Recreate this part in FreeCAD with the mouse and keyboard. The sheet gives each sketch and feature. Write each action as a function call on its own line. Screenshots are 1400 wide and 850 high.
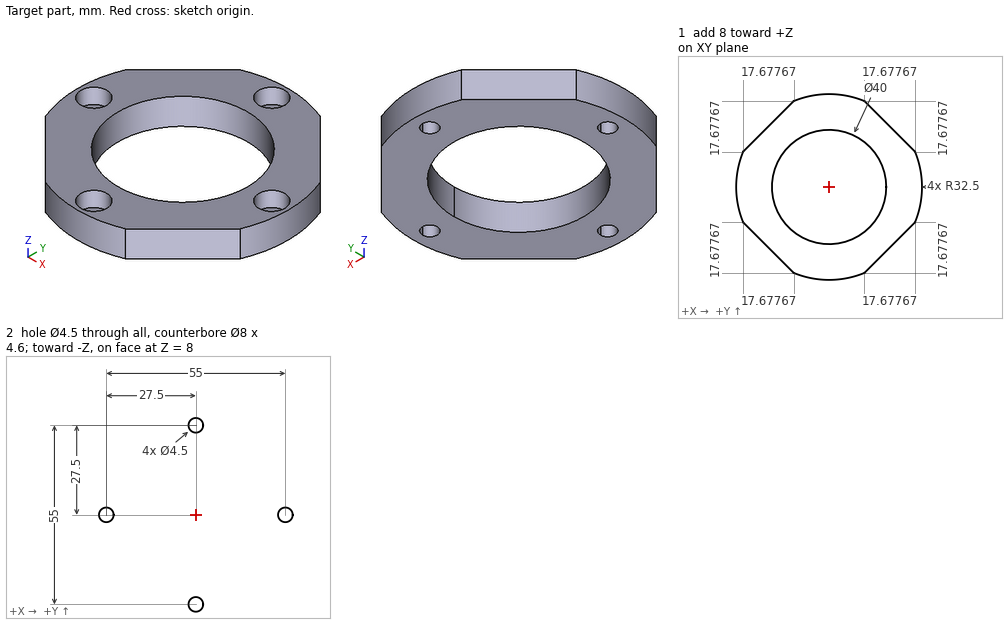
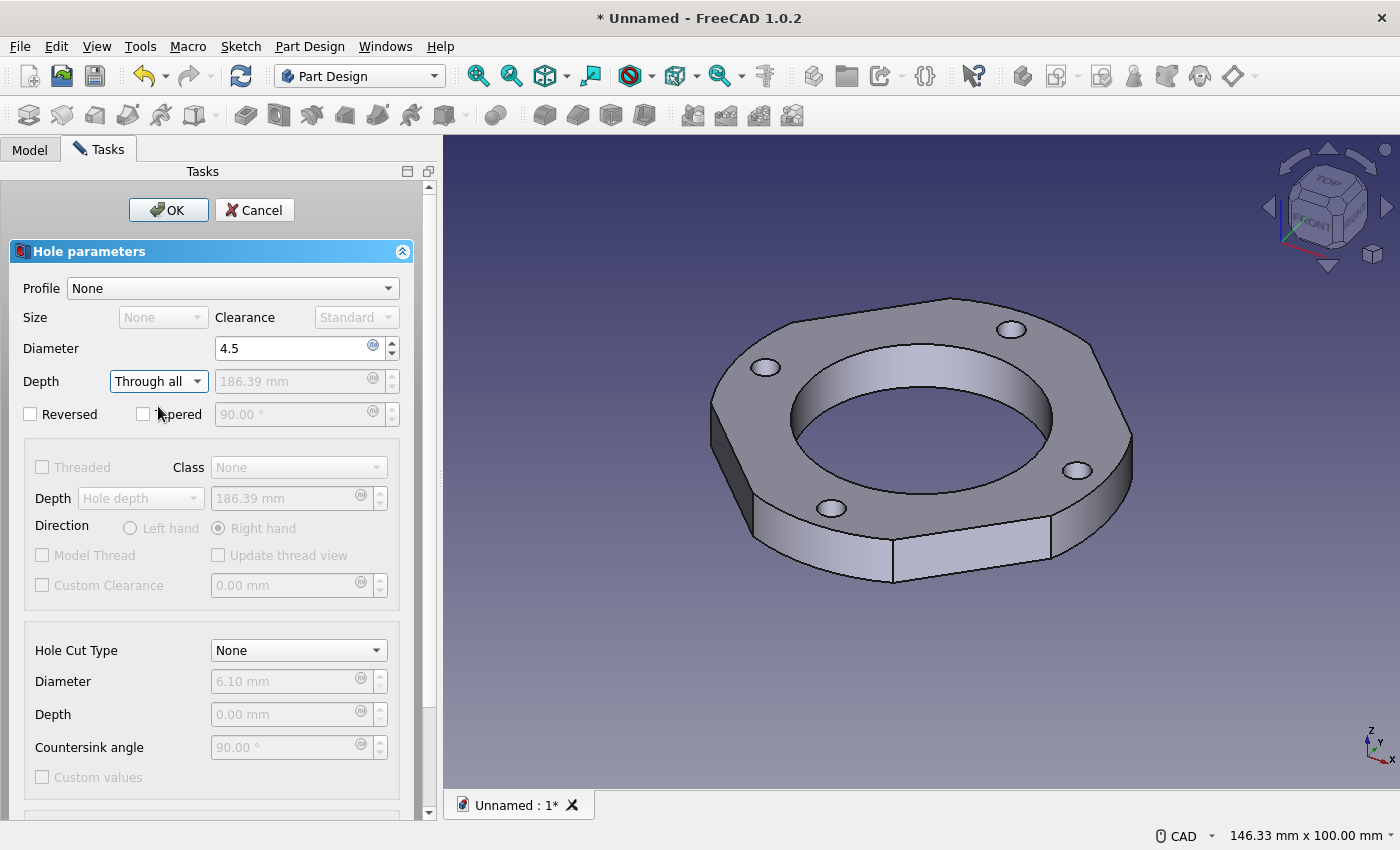
click(300, 650)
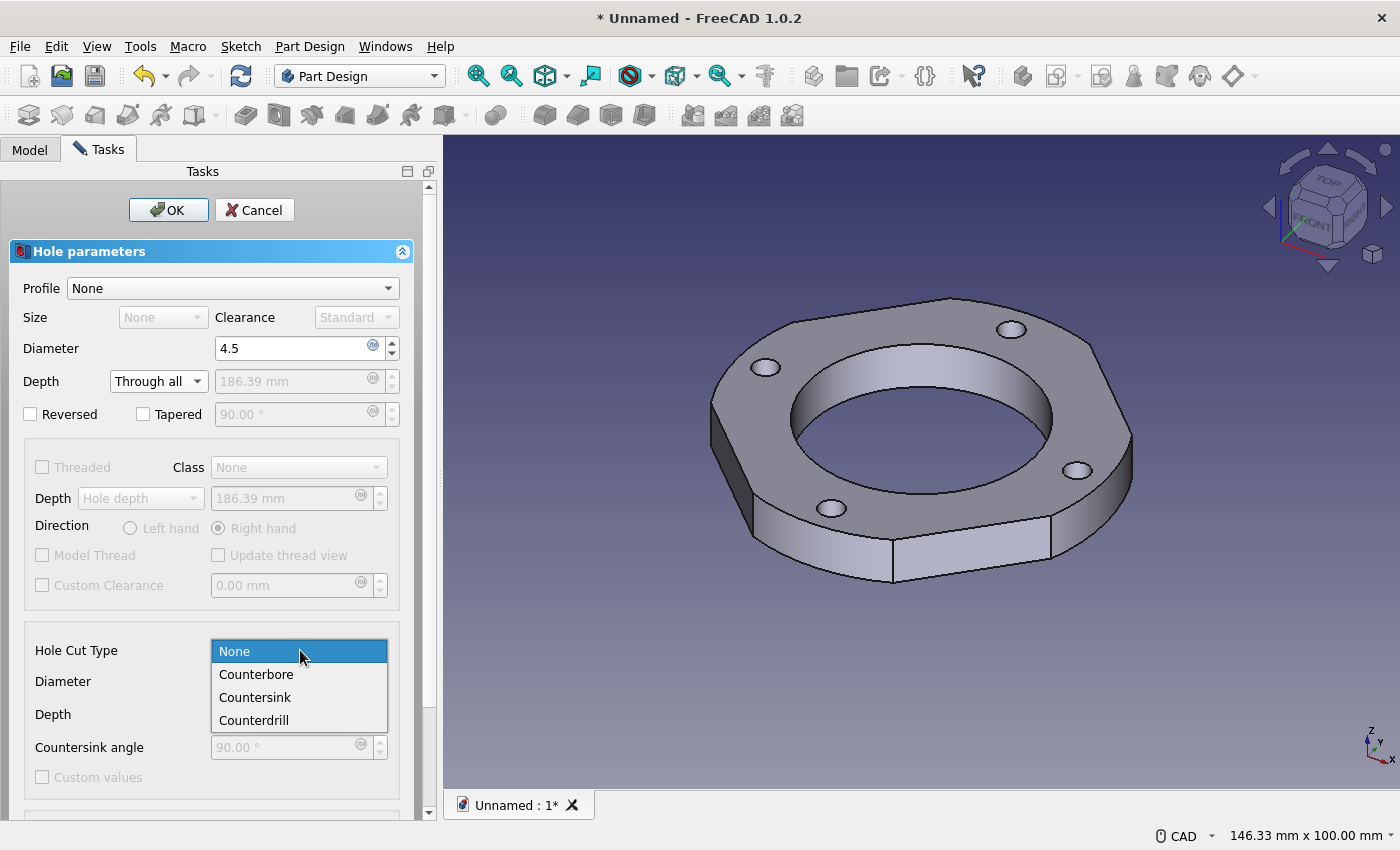
click(298, 674)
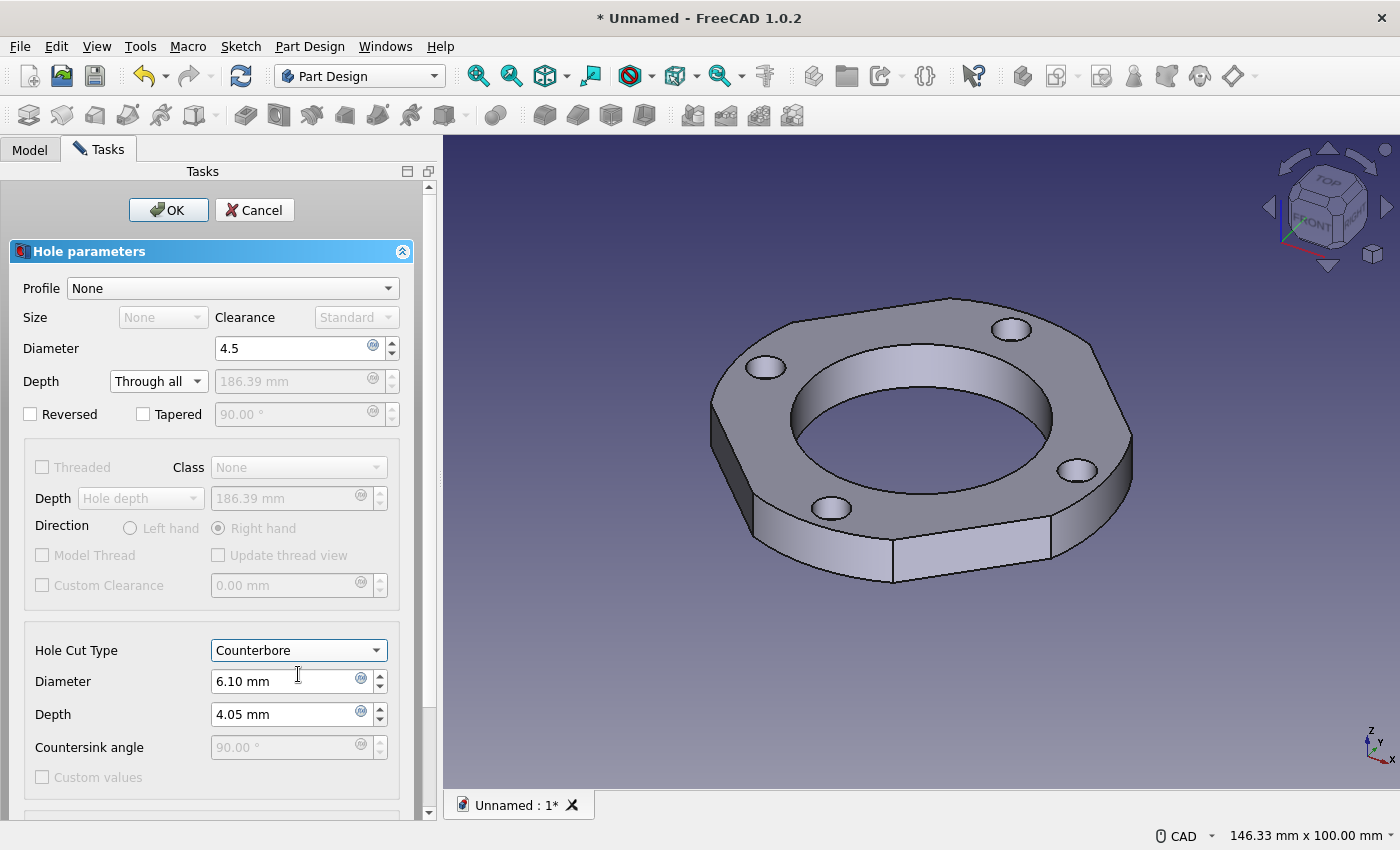
triple_click(292, 682)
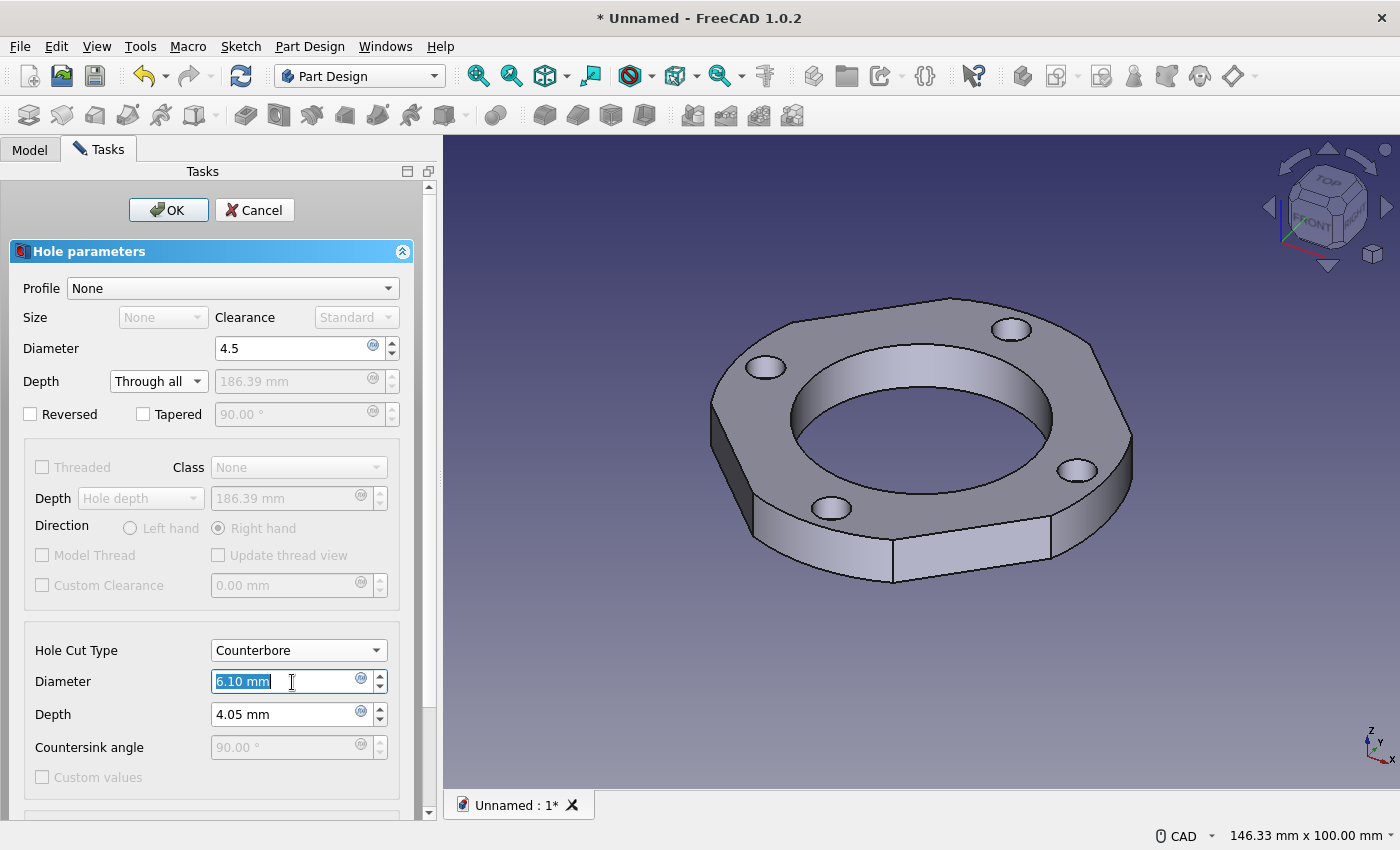
text(8)
key(Tab)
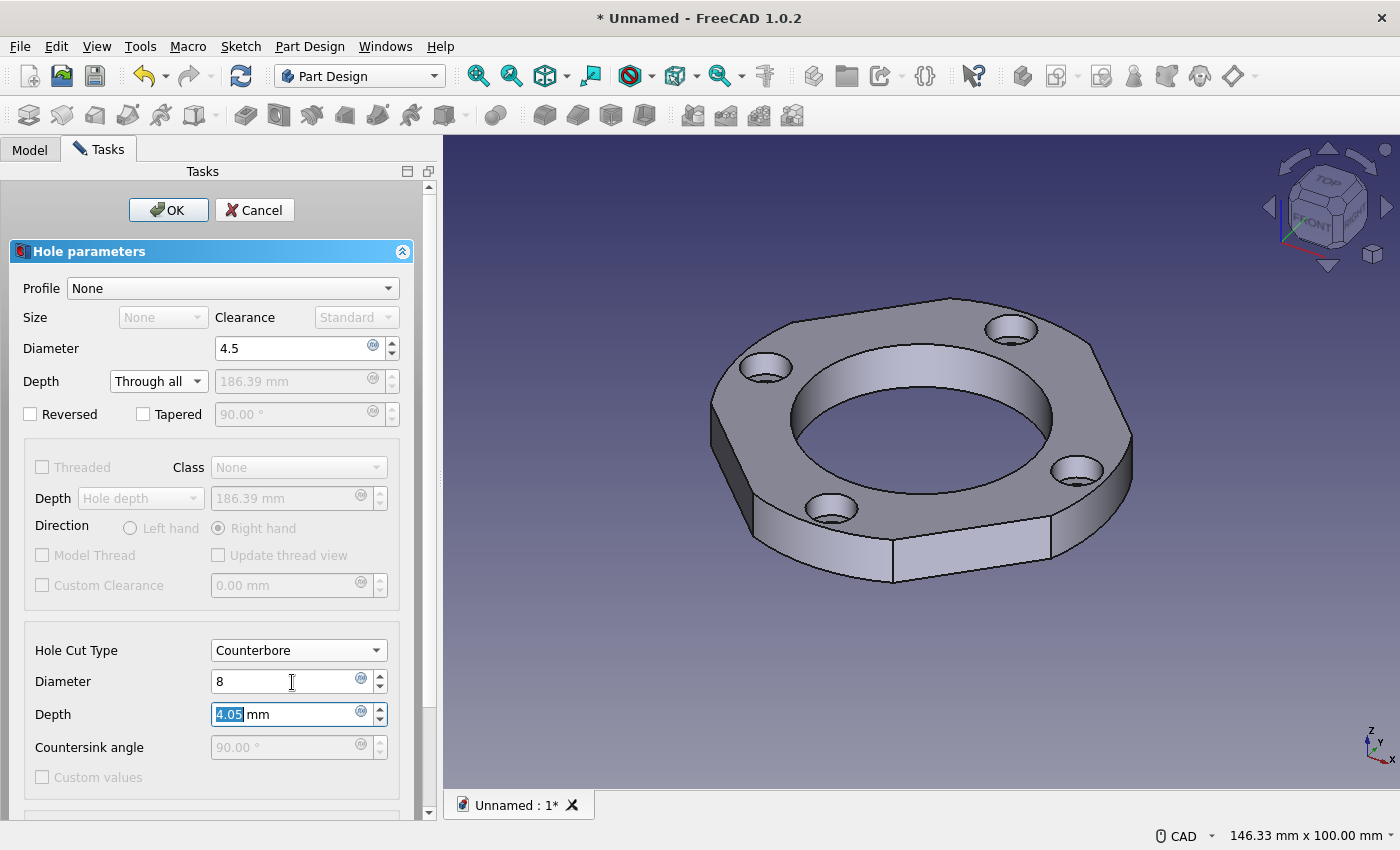
text(4.6)
key(Tab)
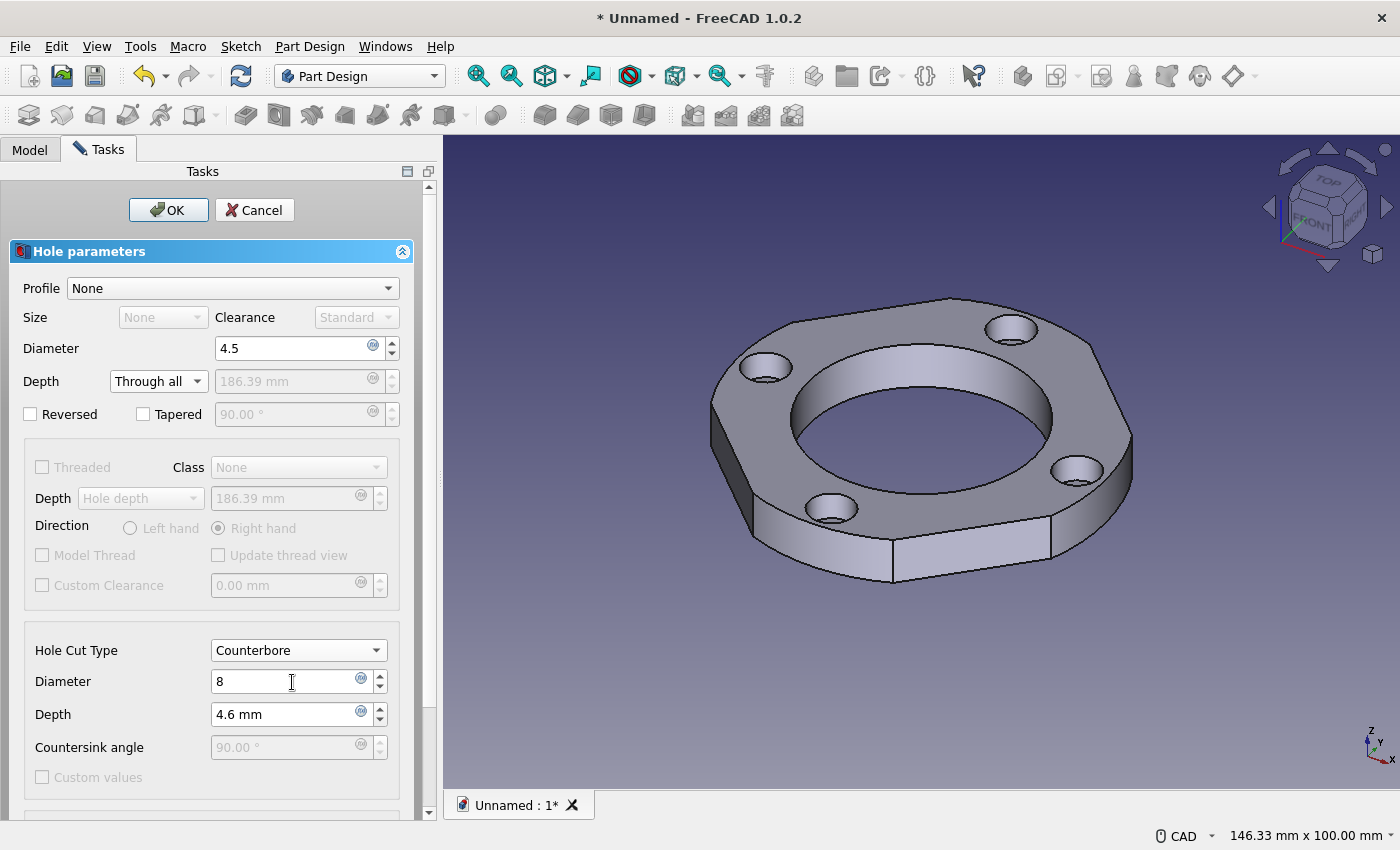
click(169, 210)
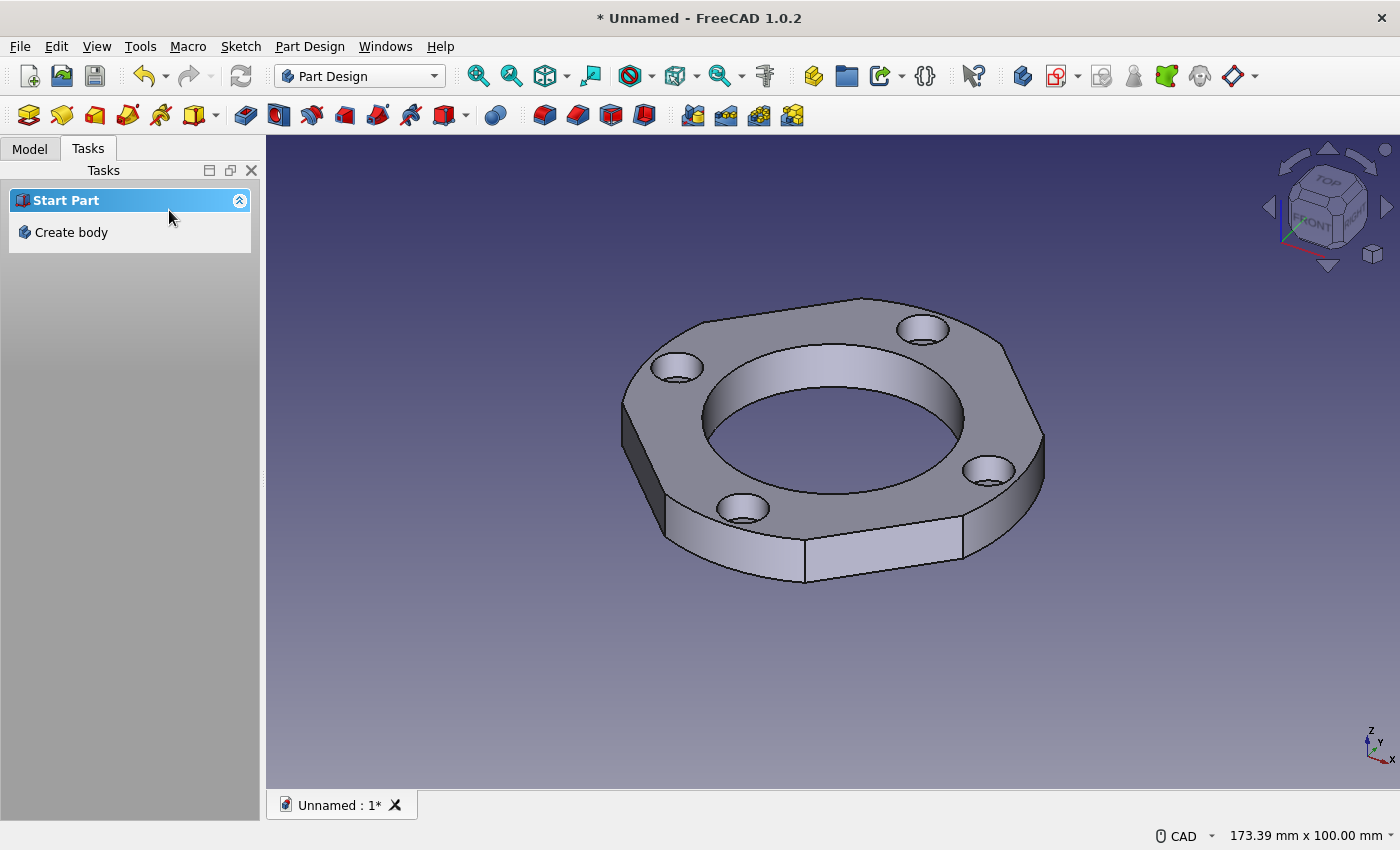
key(0)